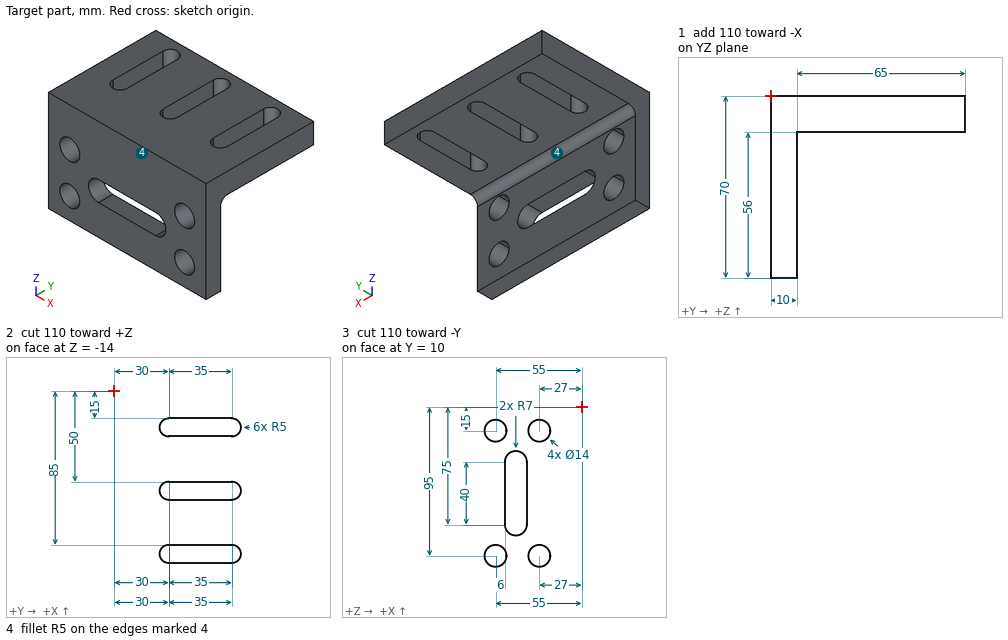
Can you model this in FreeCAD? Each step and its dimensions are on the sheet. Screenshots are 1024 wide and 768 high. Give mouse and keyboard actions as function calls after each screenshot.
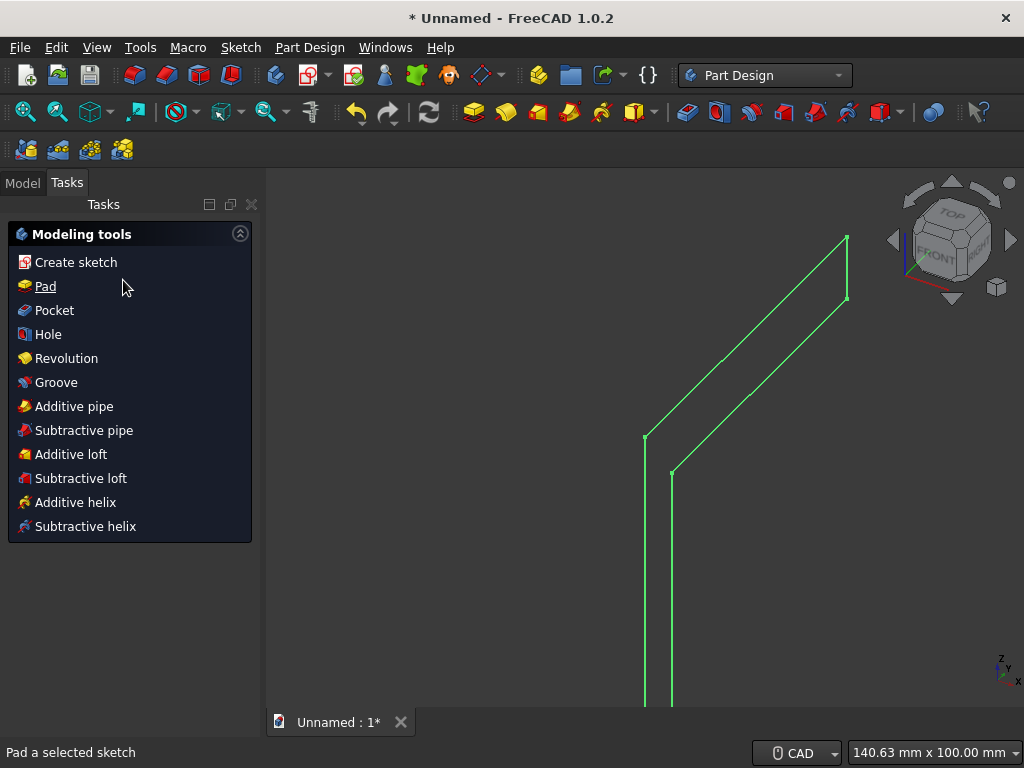
click(474, 112)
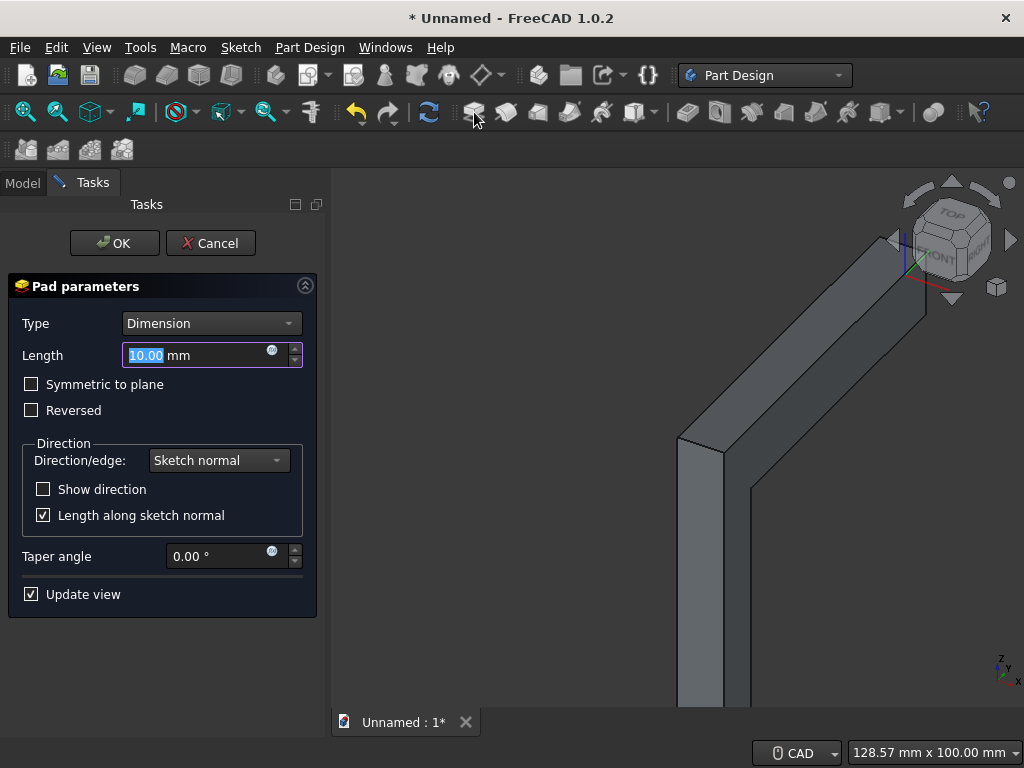
text(110)
key(Tab)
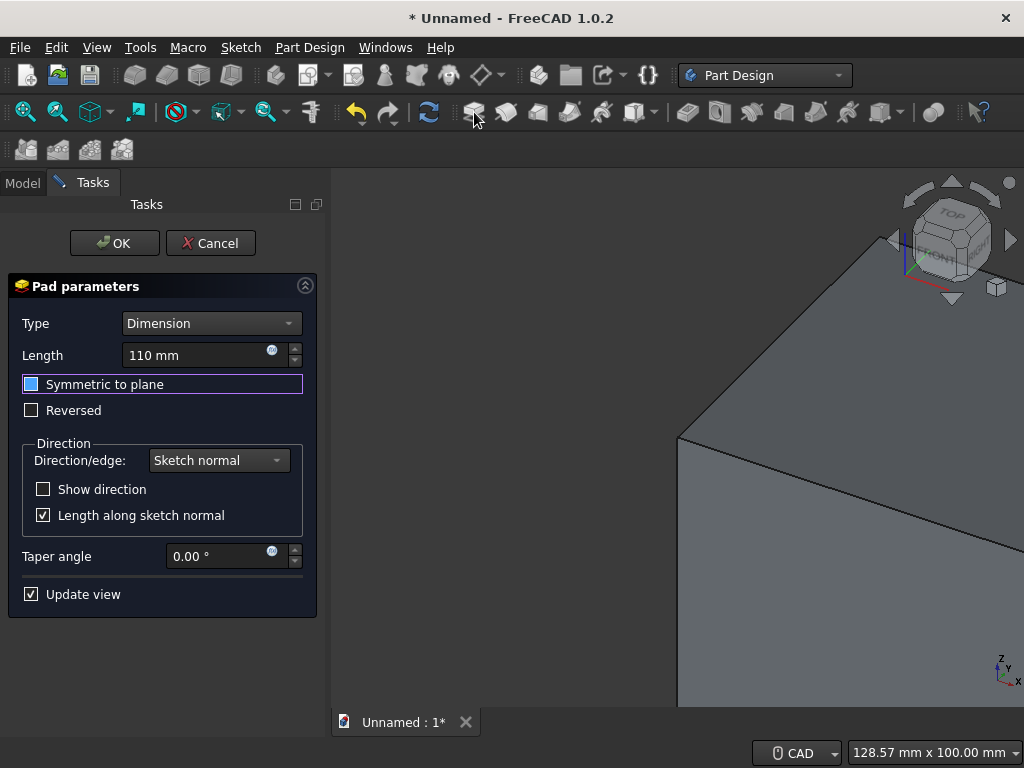
click(30, 410)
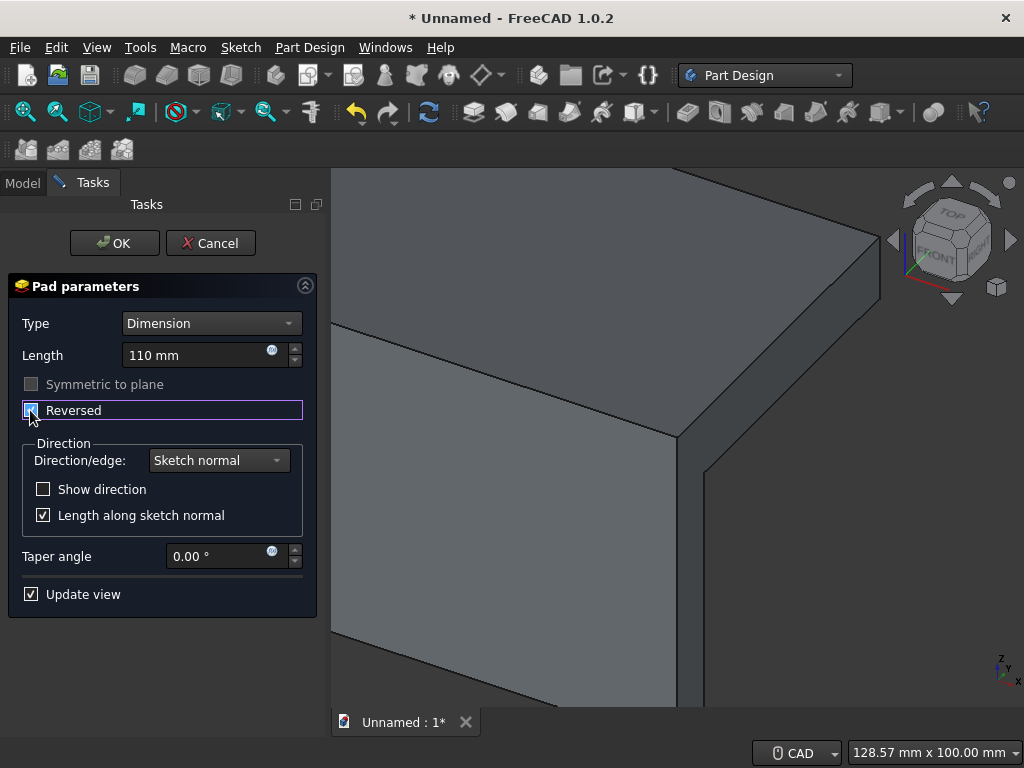
click(115, 243)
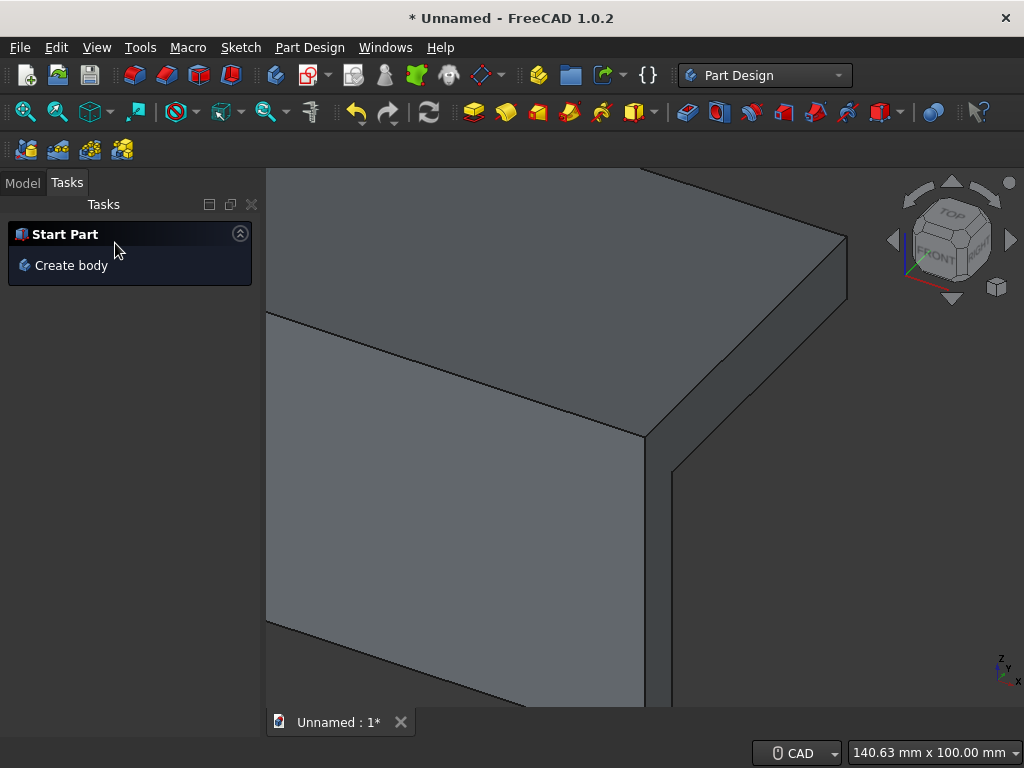
click(26, 112)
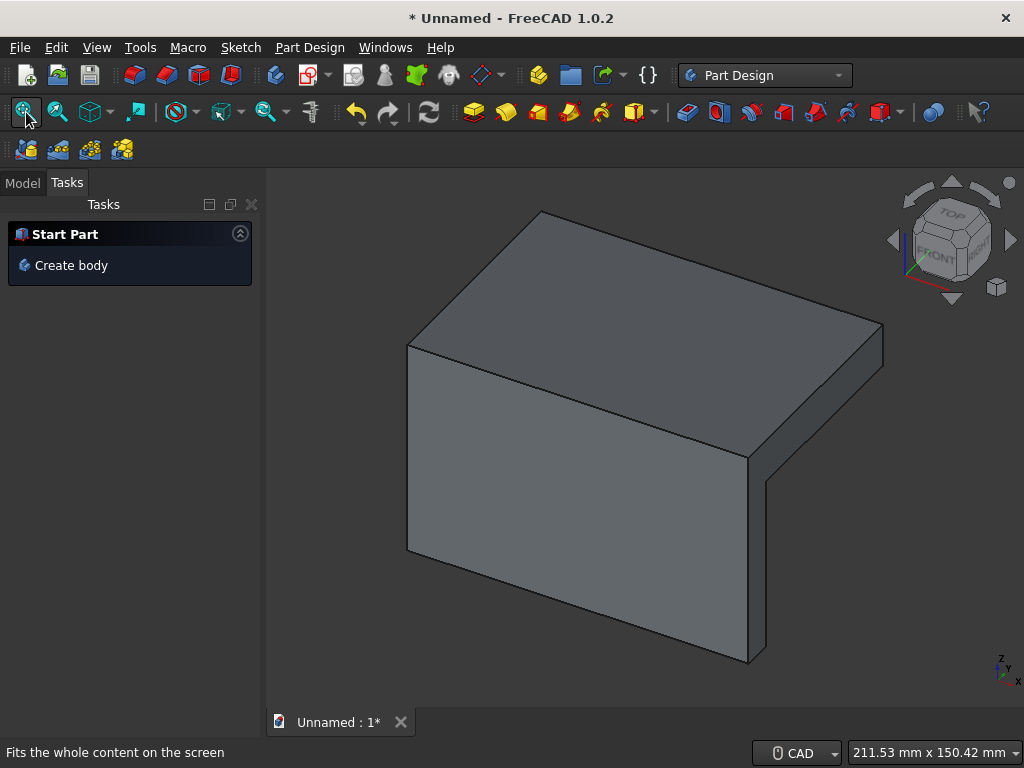
key(5)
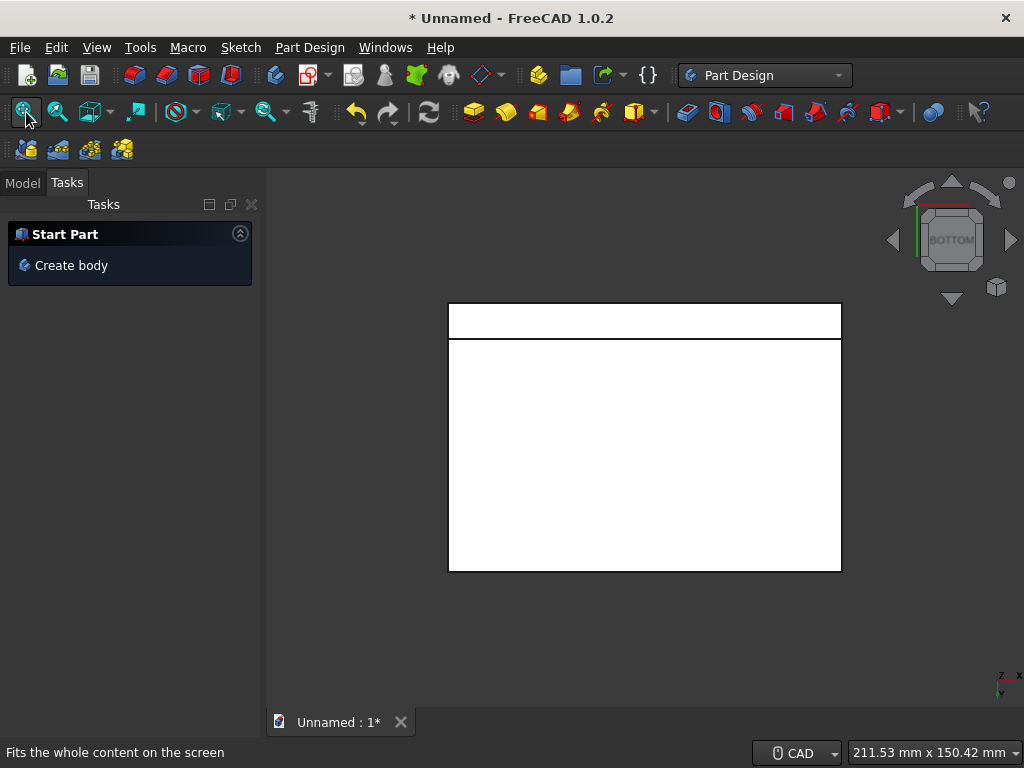
click(701, 454)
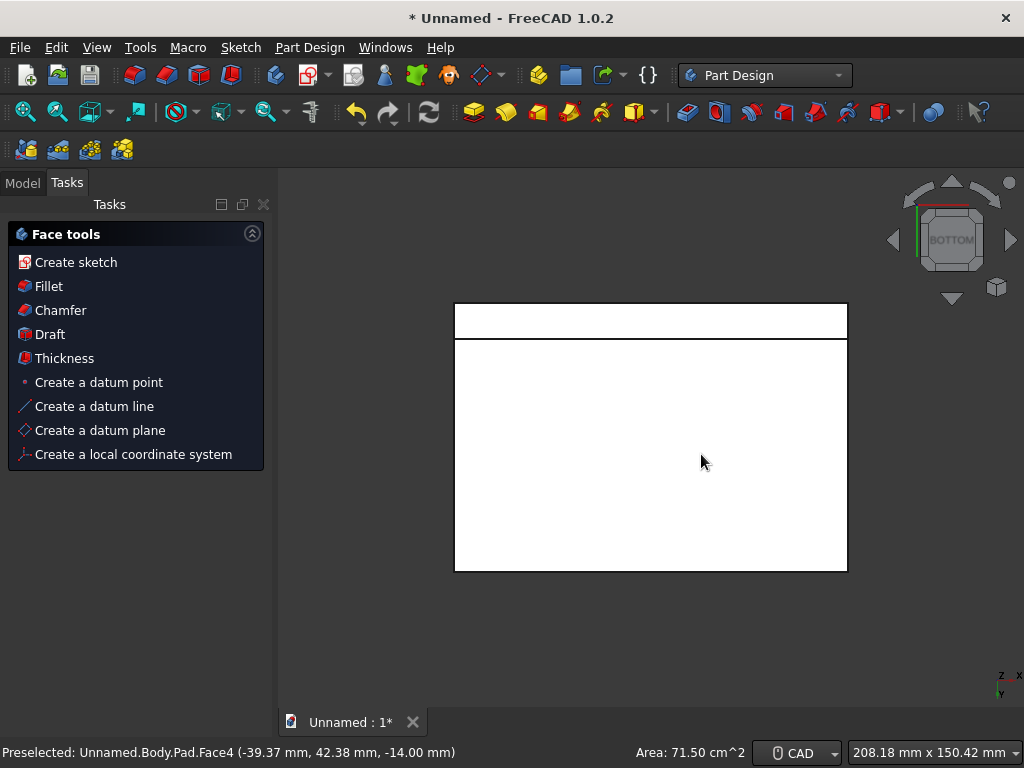
click(308, 76)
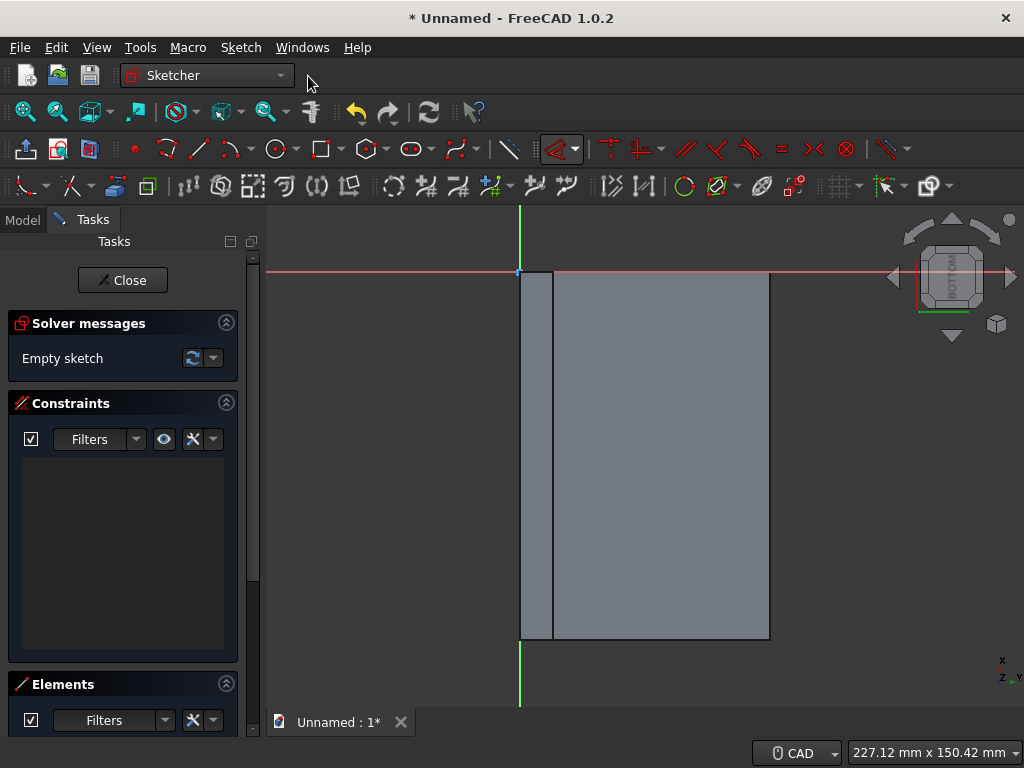
key(g)
key(s)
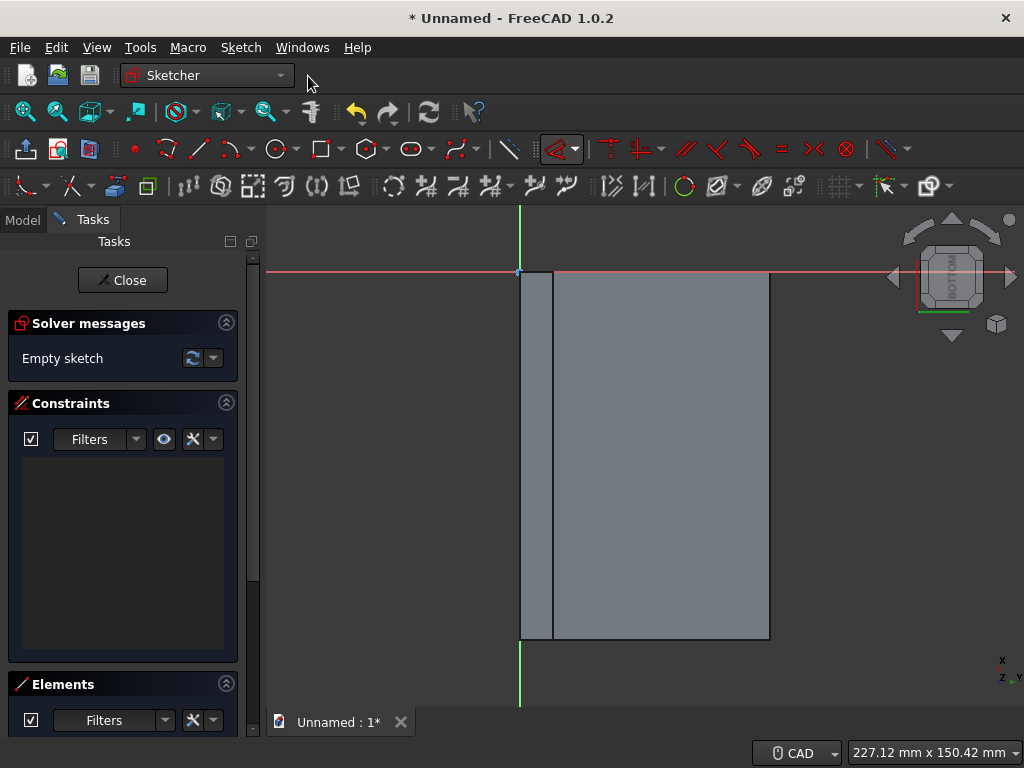
scroll(620, 339, up, 2)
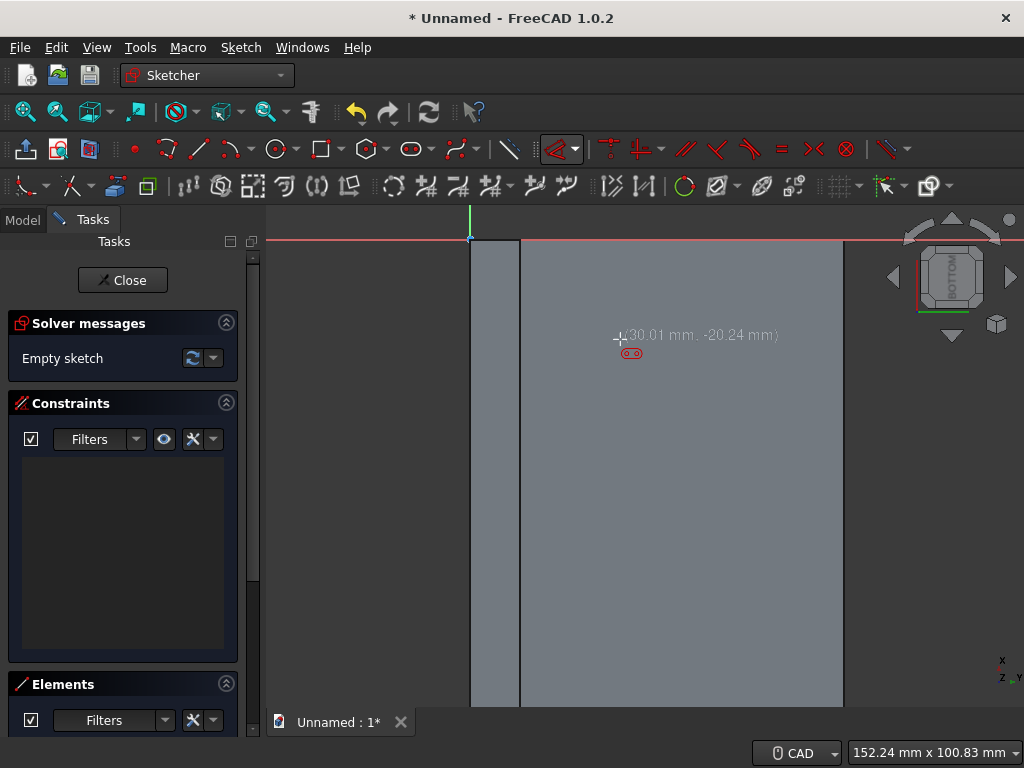
click(620, 339)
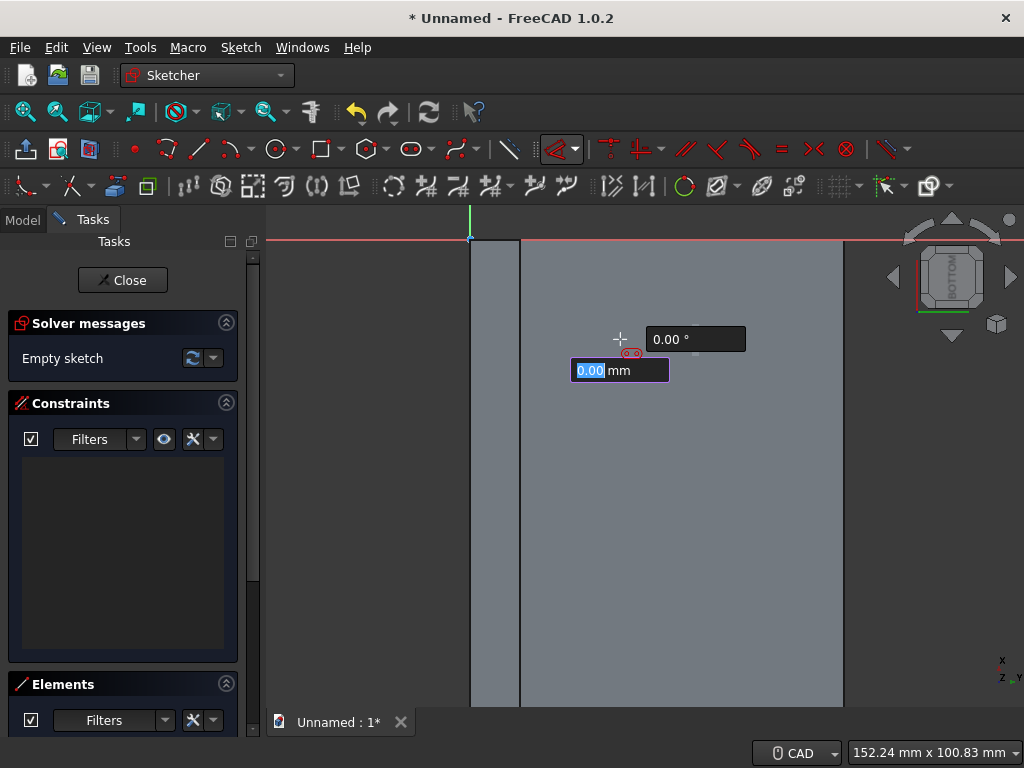
click(794, 339)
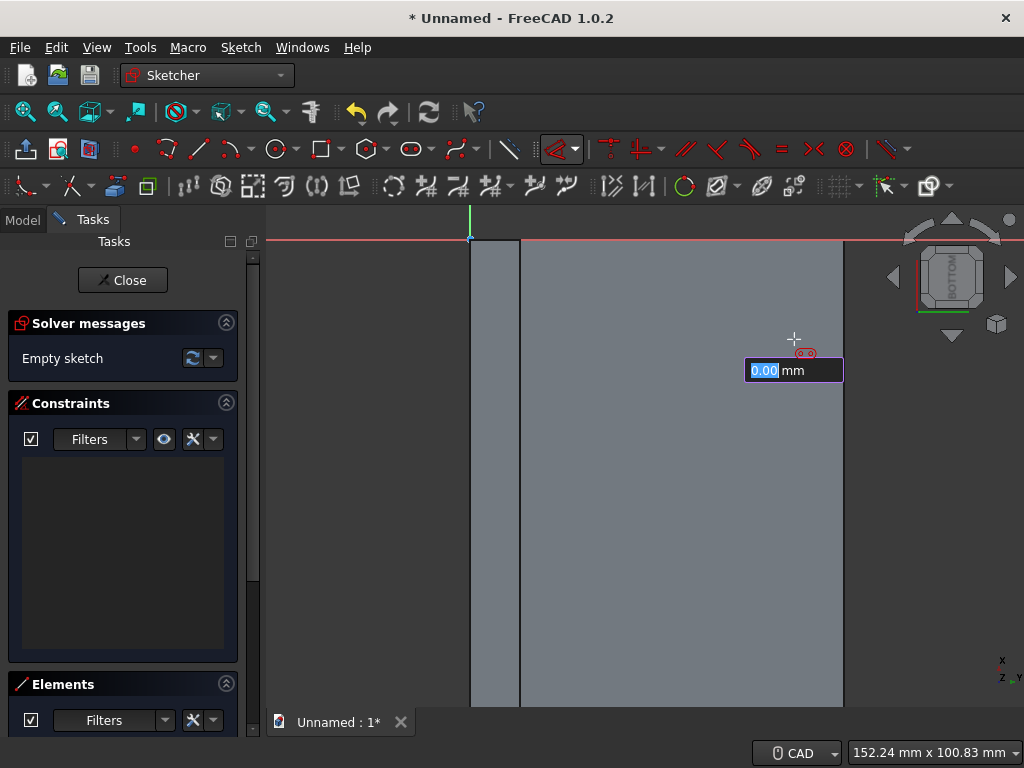
click(707, 314)